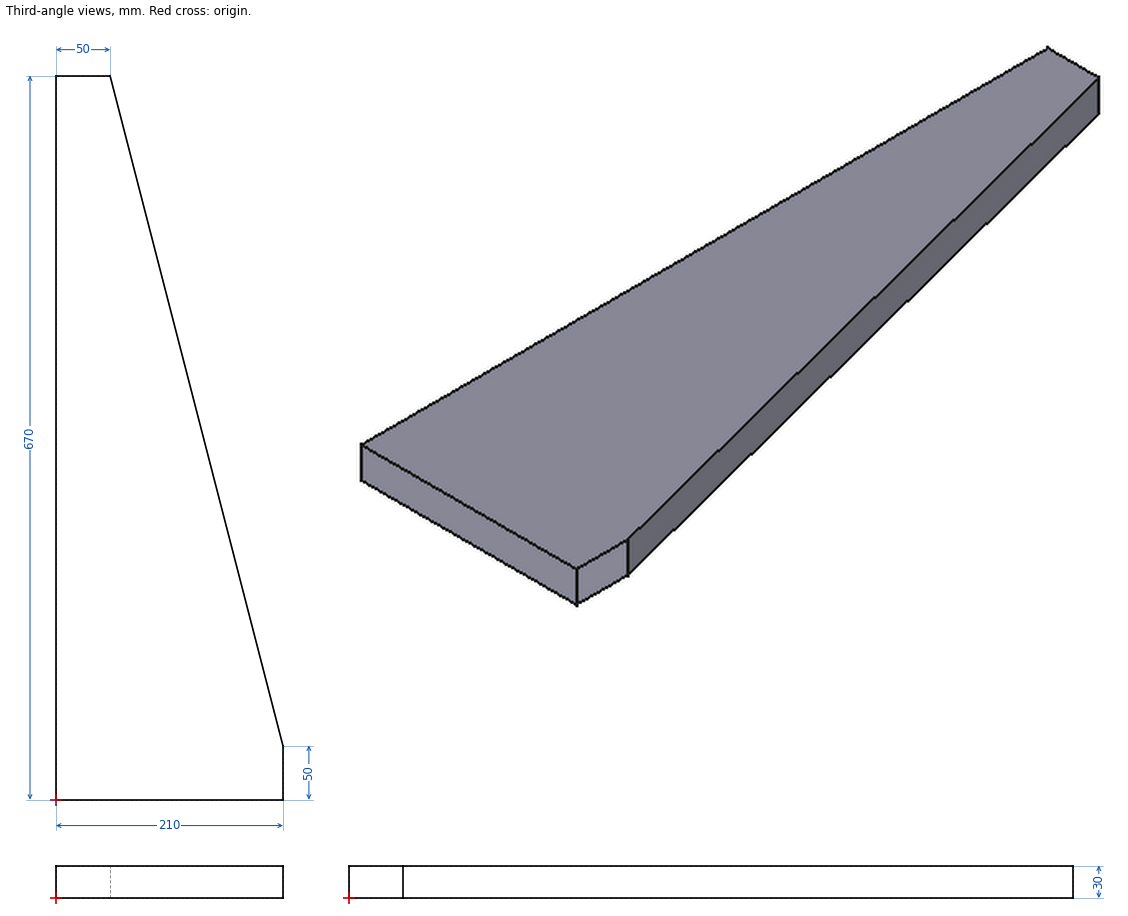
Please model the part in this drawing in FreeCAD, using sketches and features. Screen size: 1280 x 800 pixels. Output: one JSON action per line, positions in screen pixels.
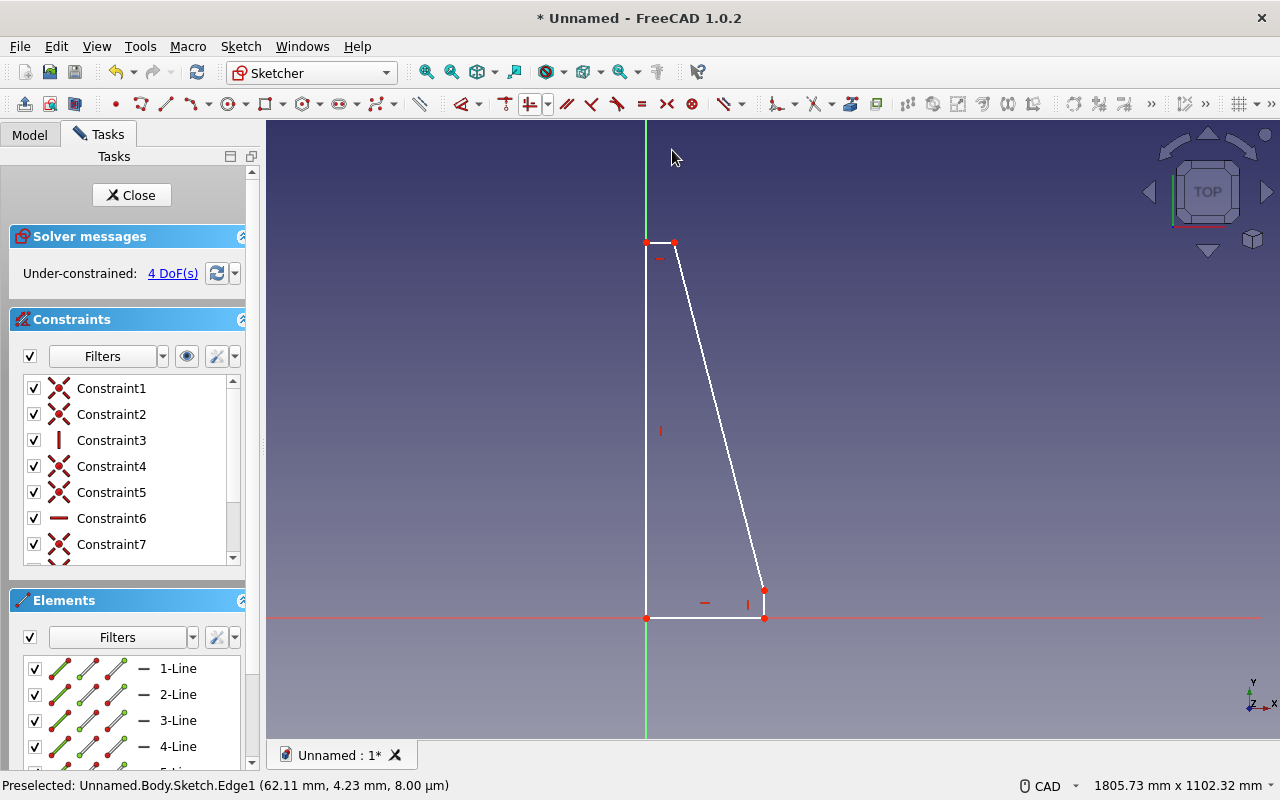
{"action": "scroll", "coordinate": [764, 607], "scroll_direction": "up", "scroll_amount": 2}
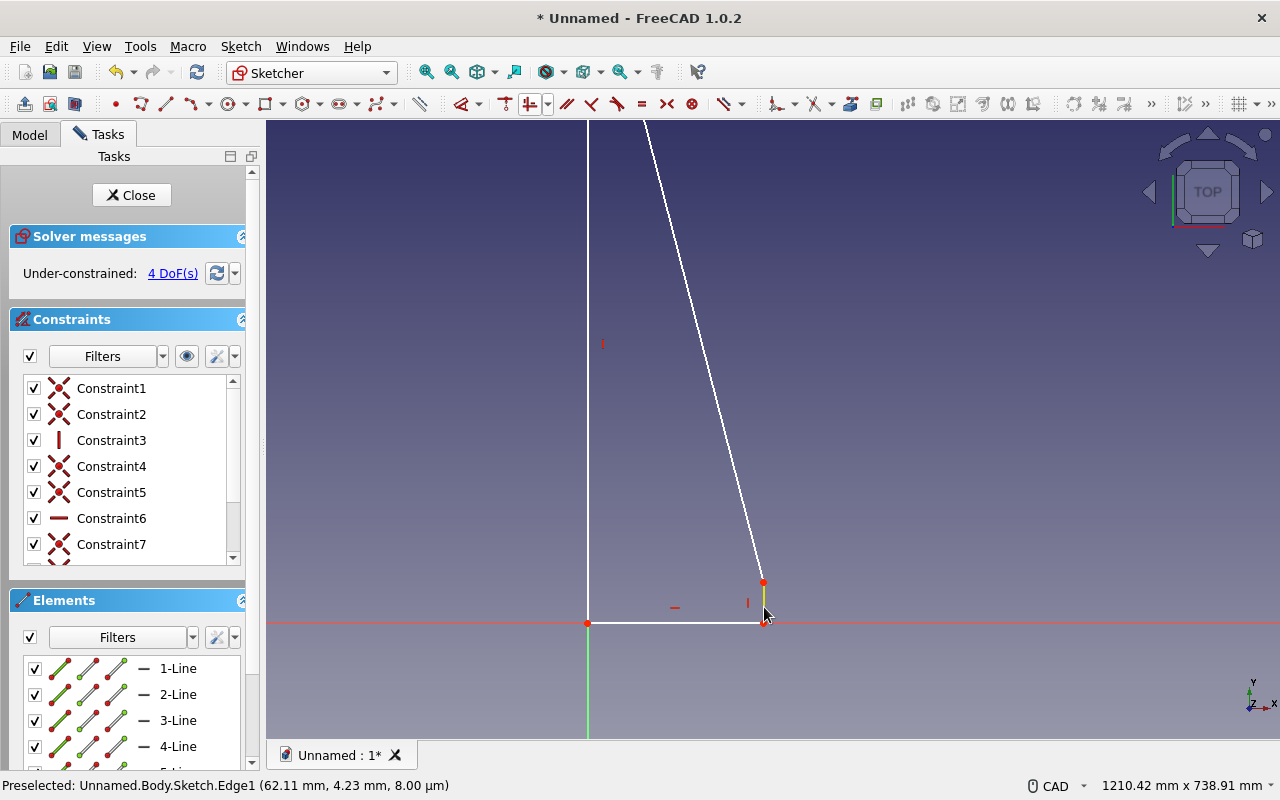
{"action": "left_click", "coordinate": [764, 607]}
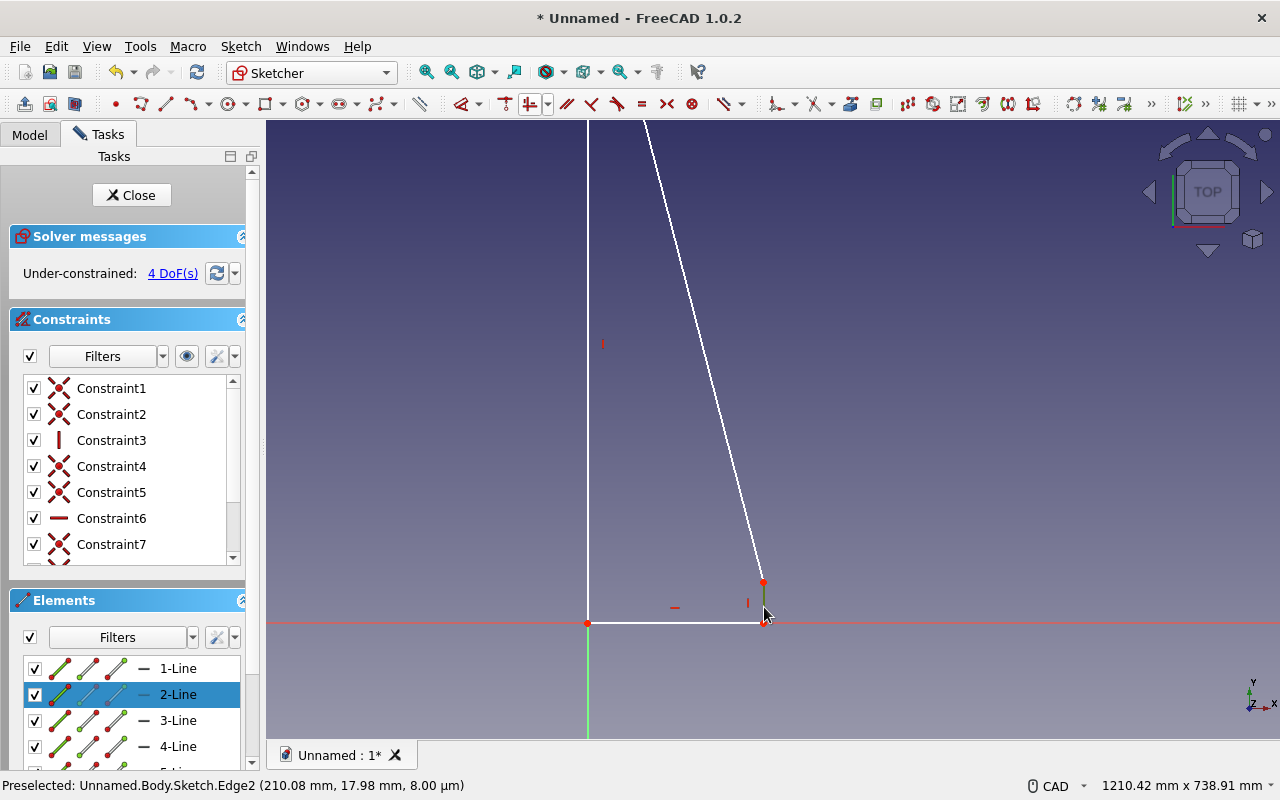
{"action": "left_click", "coordinate": [478, 104]}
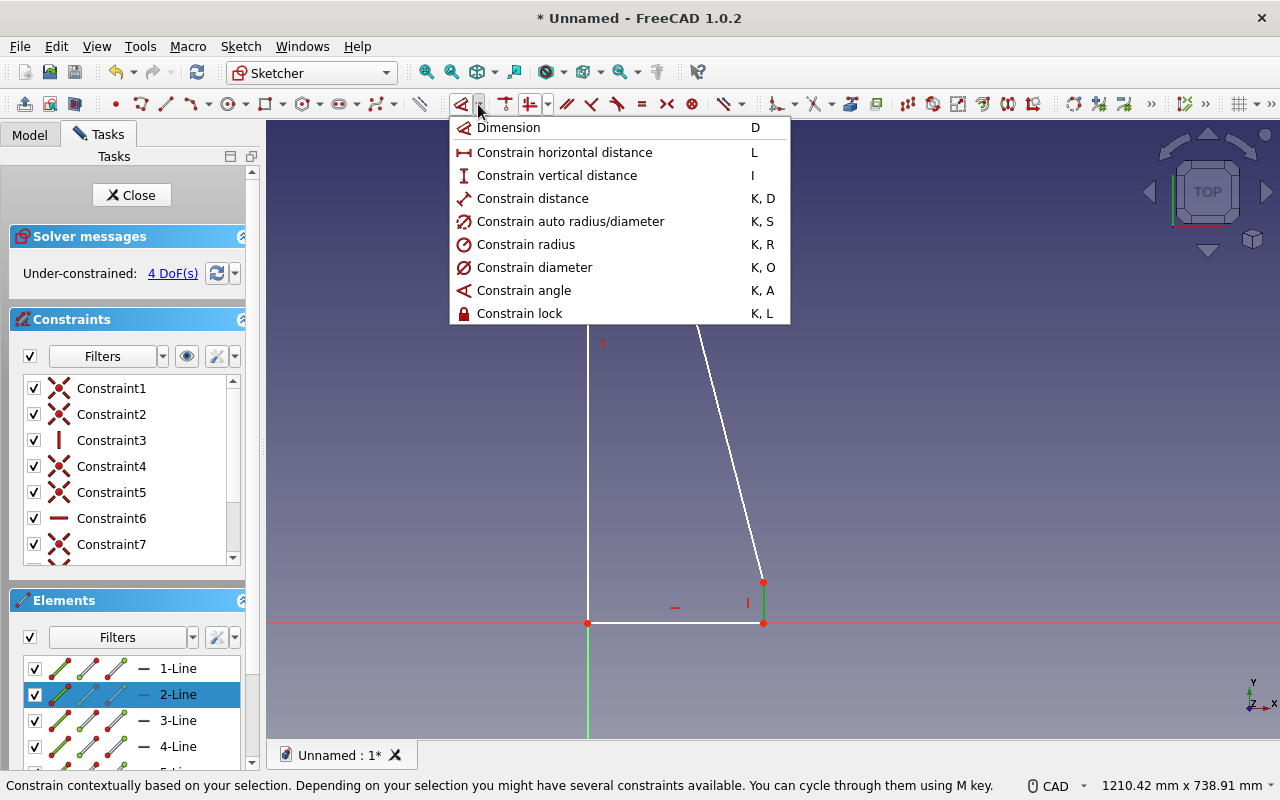
{"action": "left_click", "coordinate": [620, 176]}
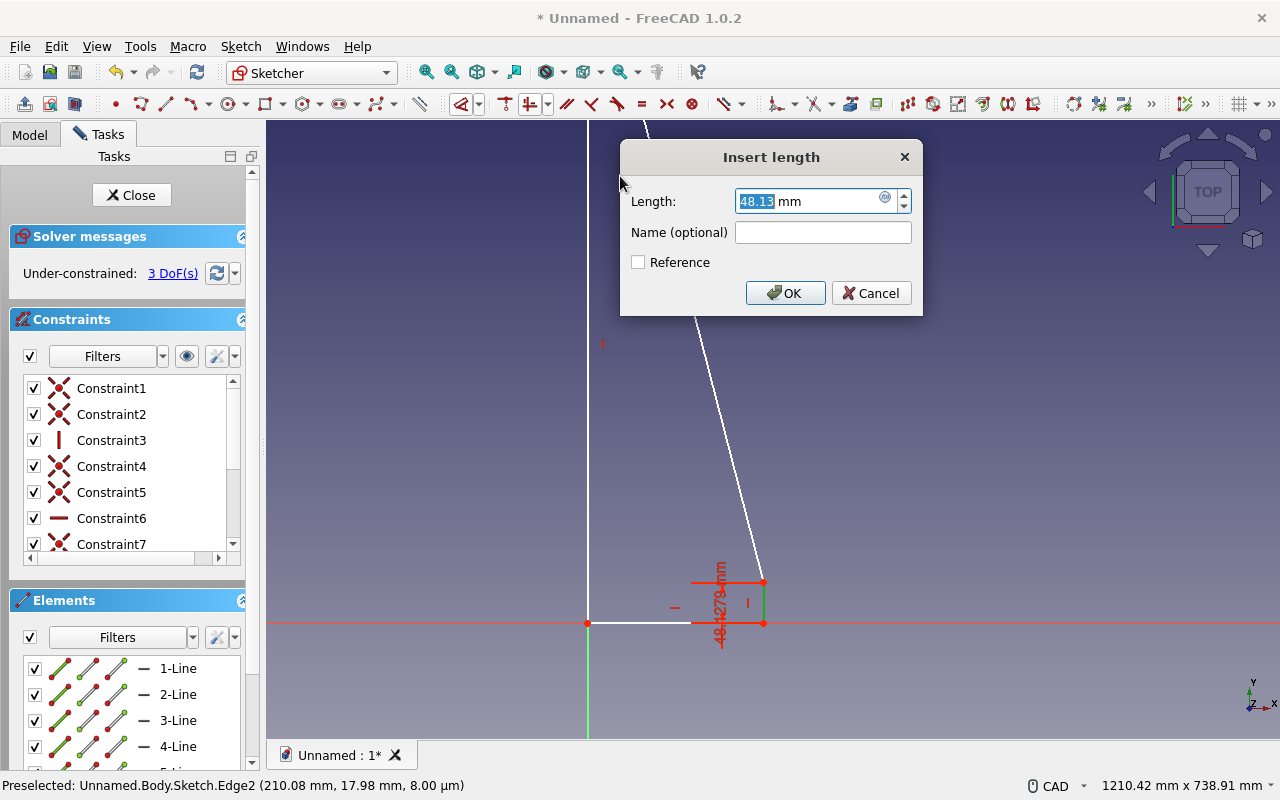
{"action": "type", "text": "50"}
{"action": "key", "text": "Return"}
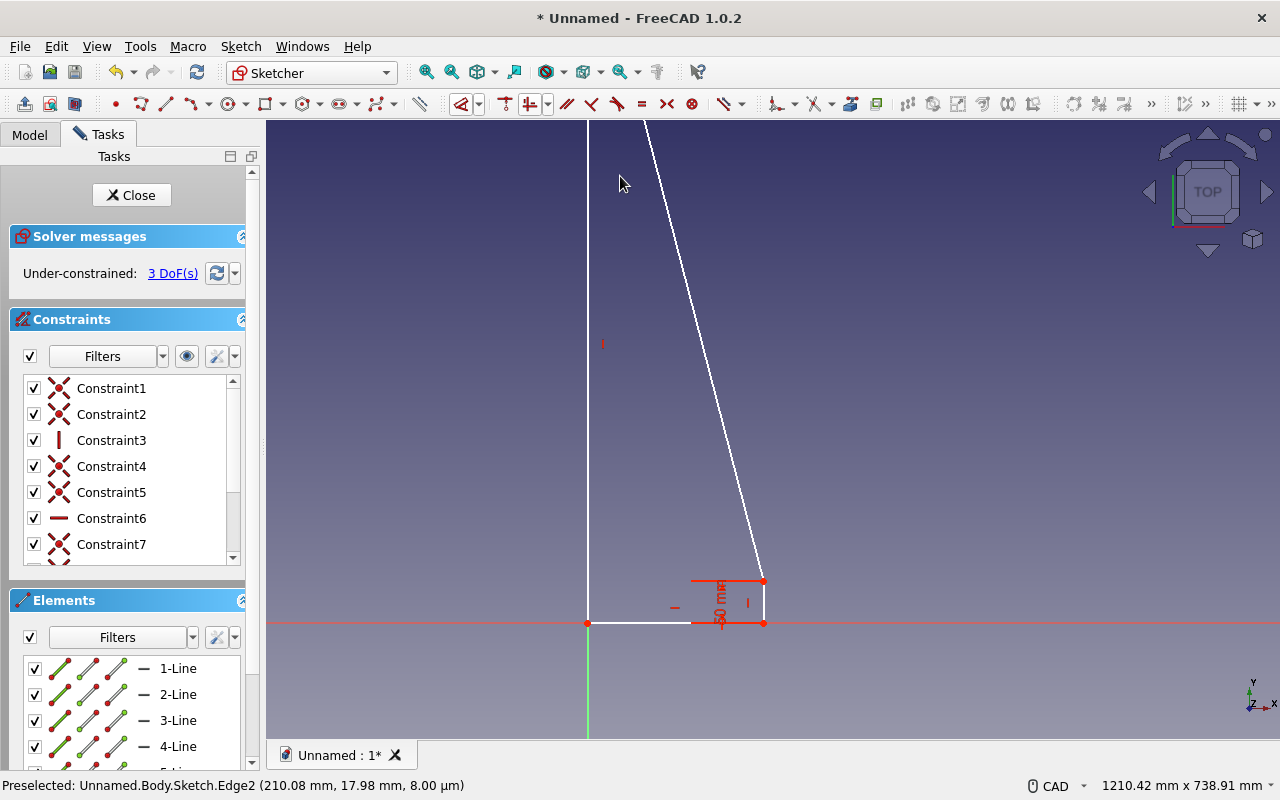
{"action": "scroll", "coordinate": [763, 607], "scroll_direction": "down", "scroll_amount": 2}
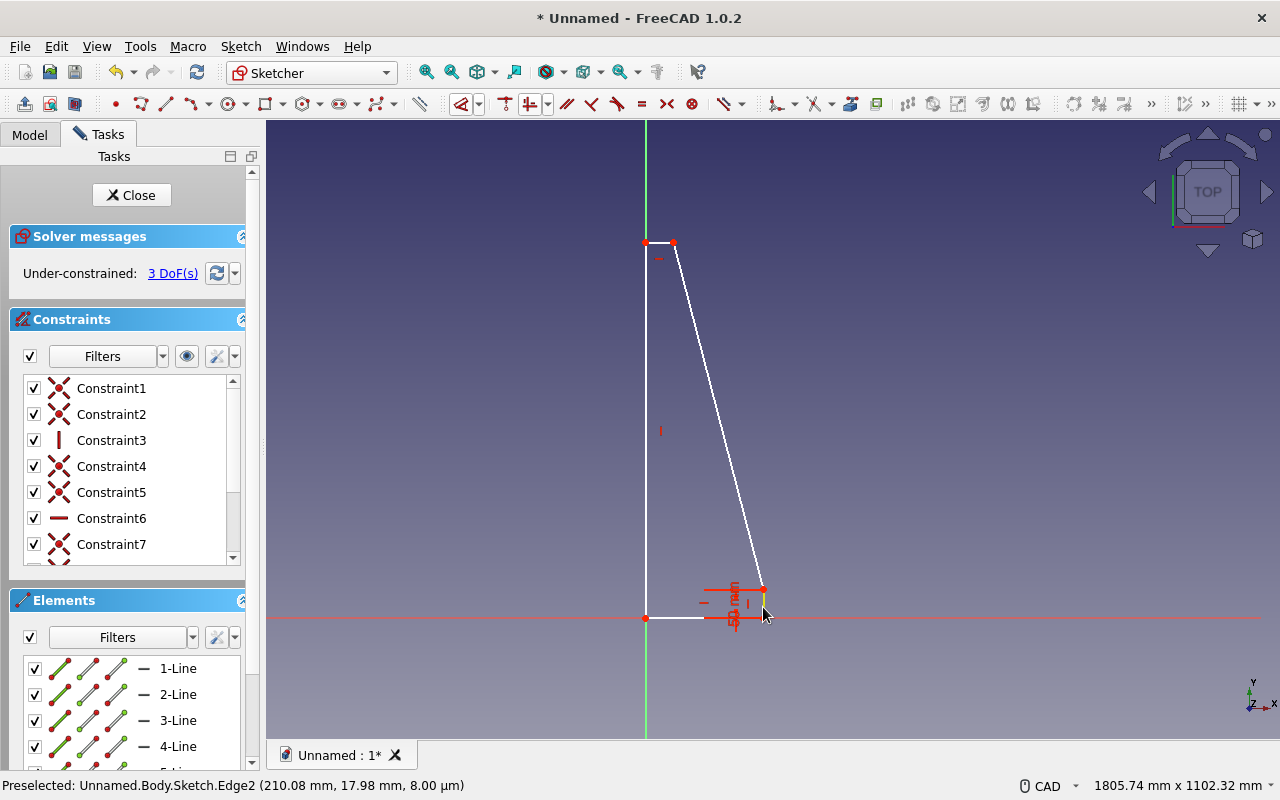
{"action": "scroll", "coordinate": [665, 243], "scroll_direction": "up", "scroll_amount": 3}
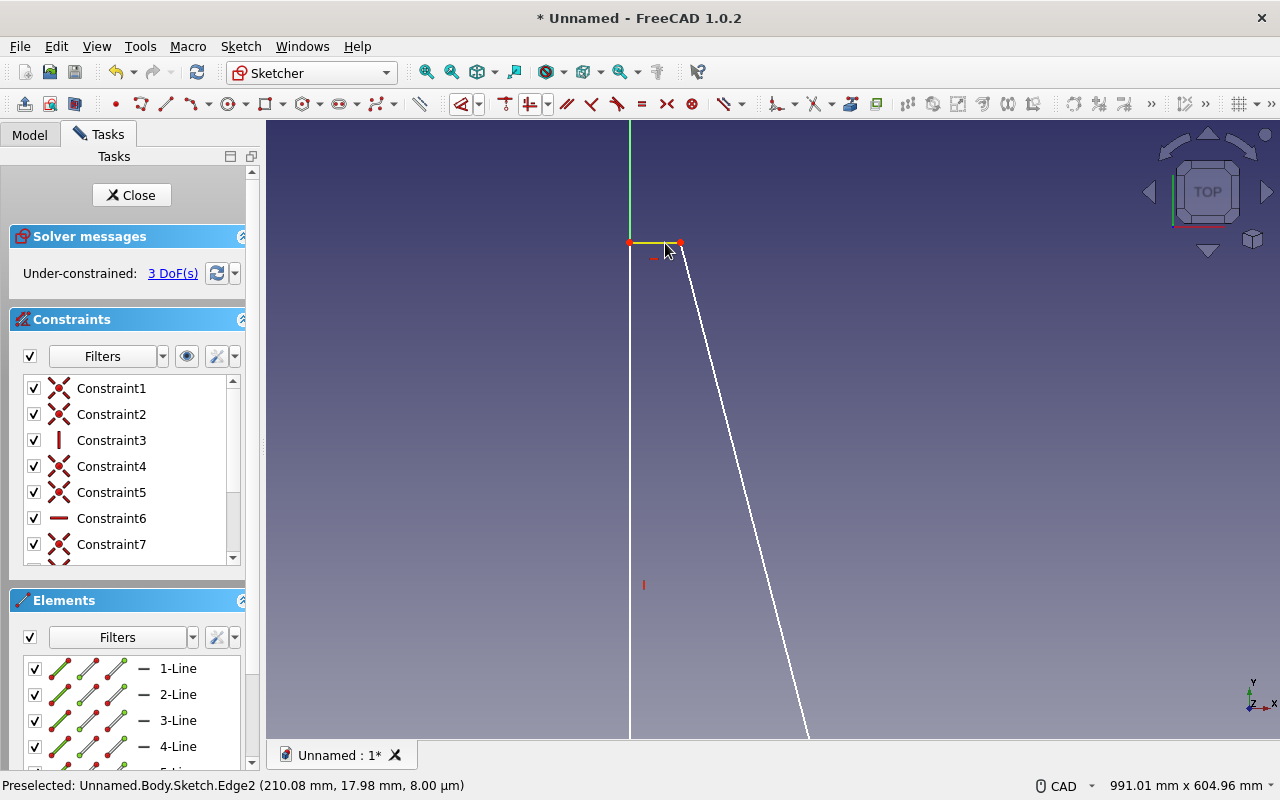
{"action": "left_click", "coordinate": [665, 243]}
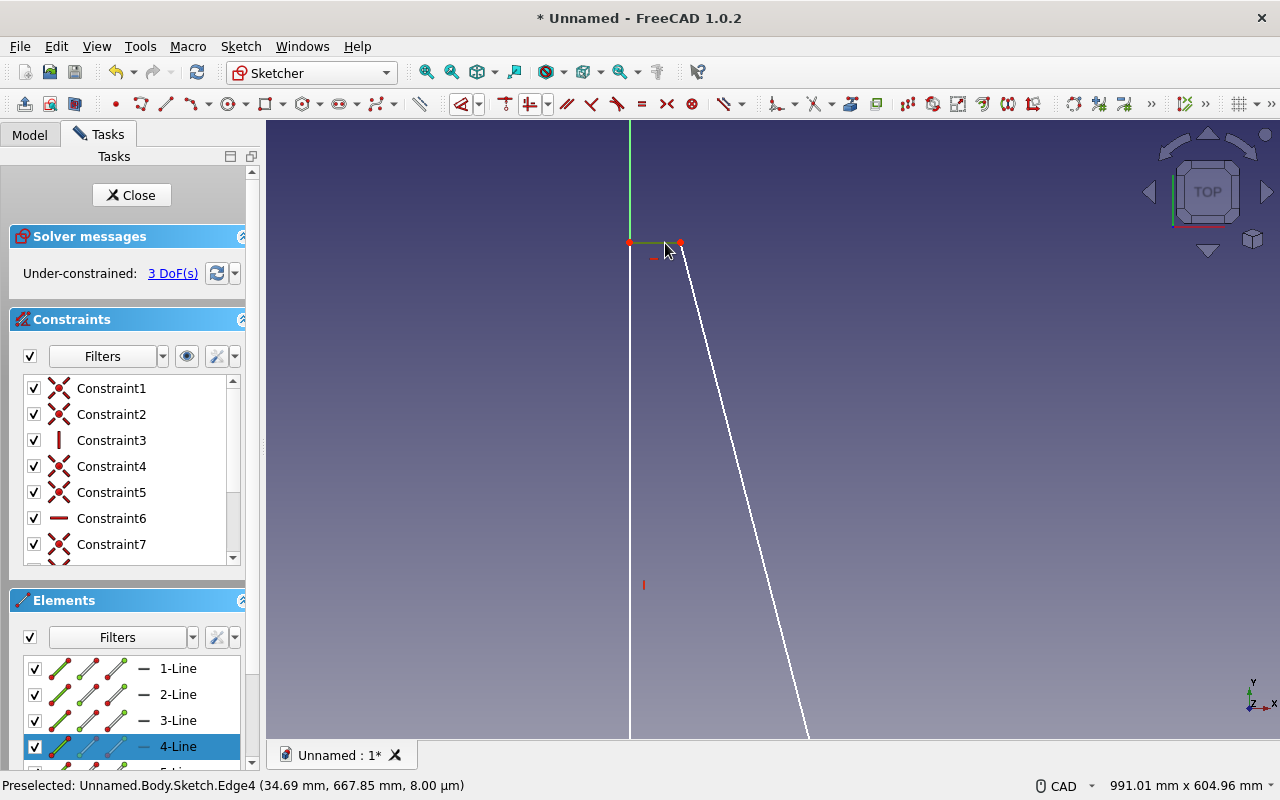
{"action": "key", "text": "l"}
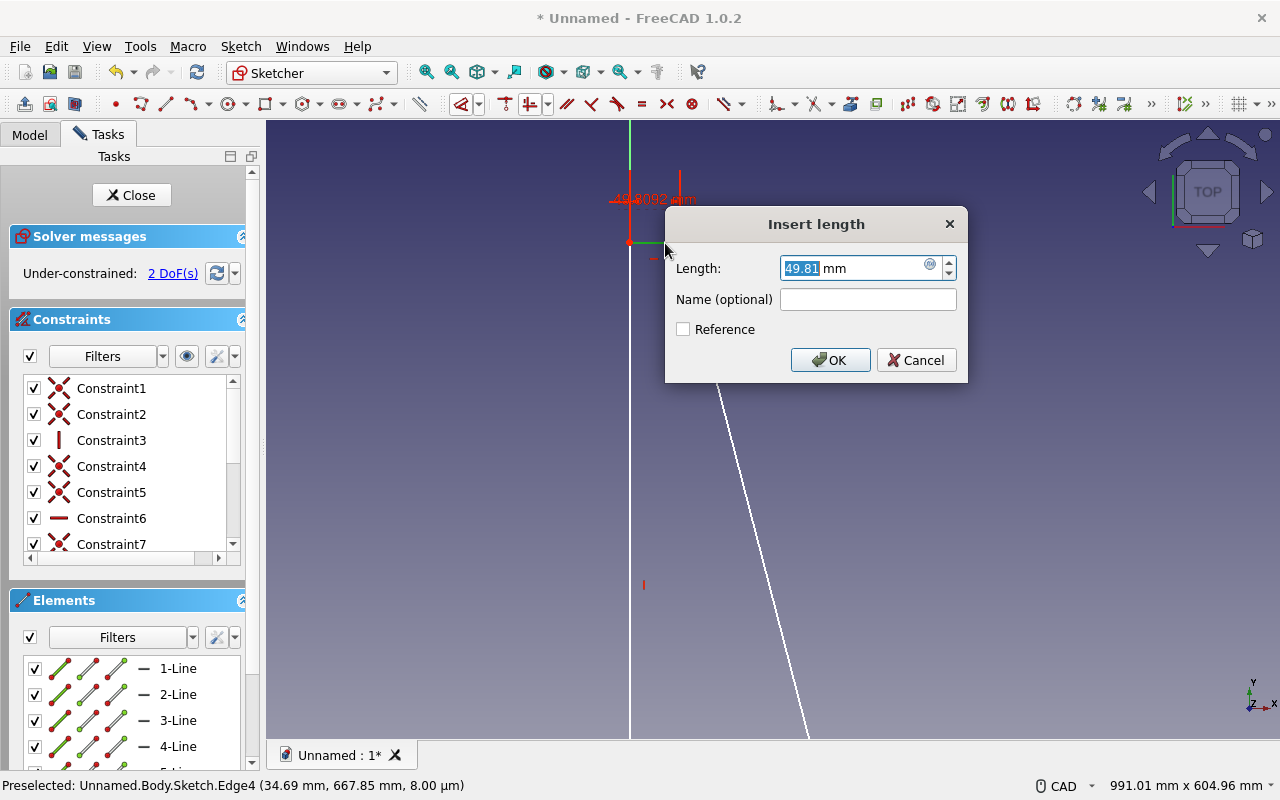
{"action": "type", "text": "50"}
{"action": "key", "text": "Return"}